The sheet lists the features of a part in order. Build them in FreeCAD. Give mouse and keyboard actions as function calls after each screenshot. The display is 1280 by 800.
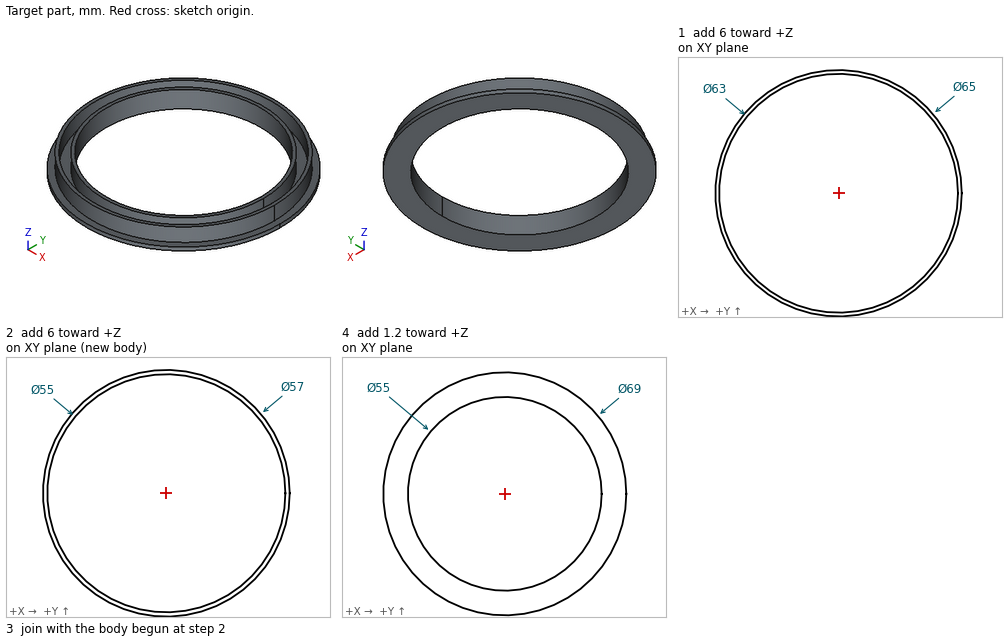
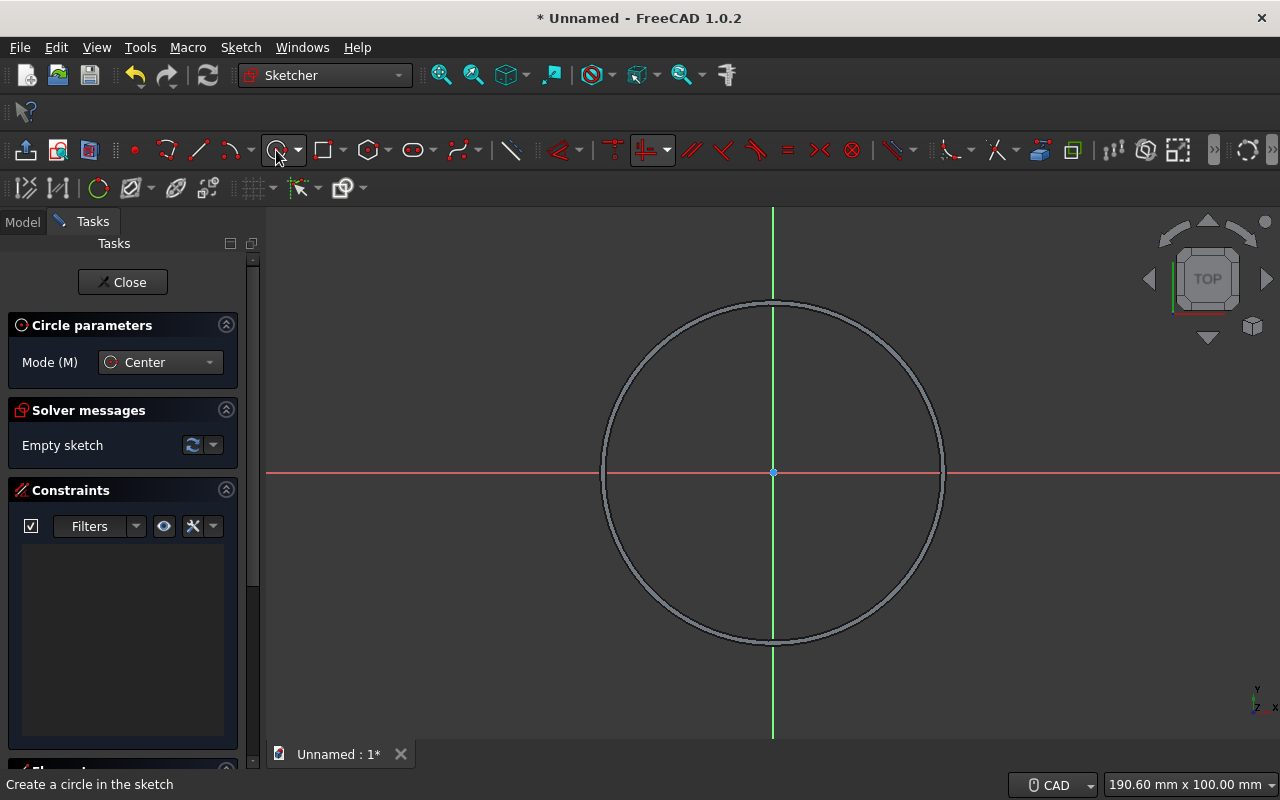
click(773, 473)
move(880, 366)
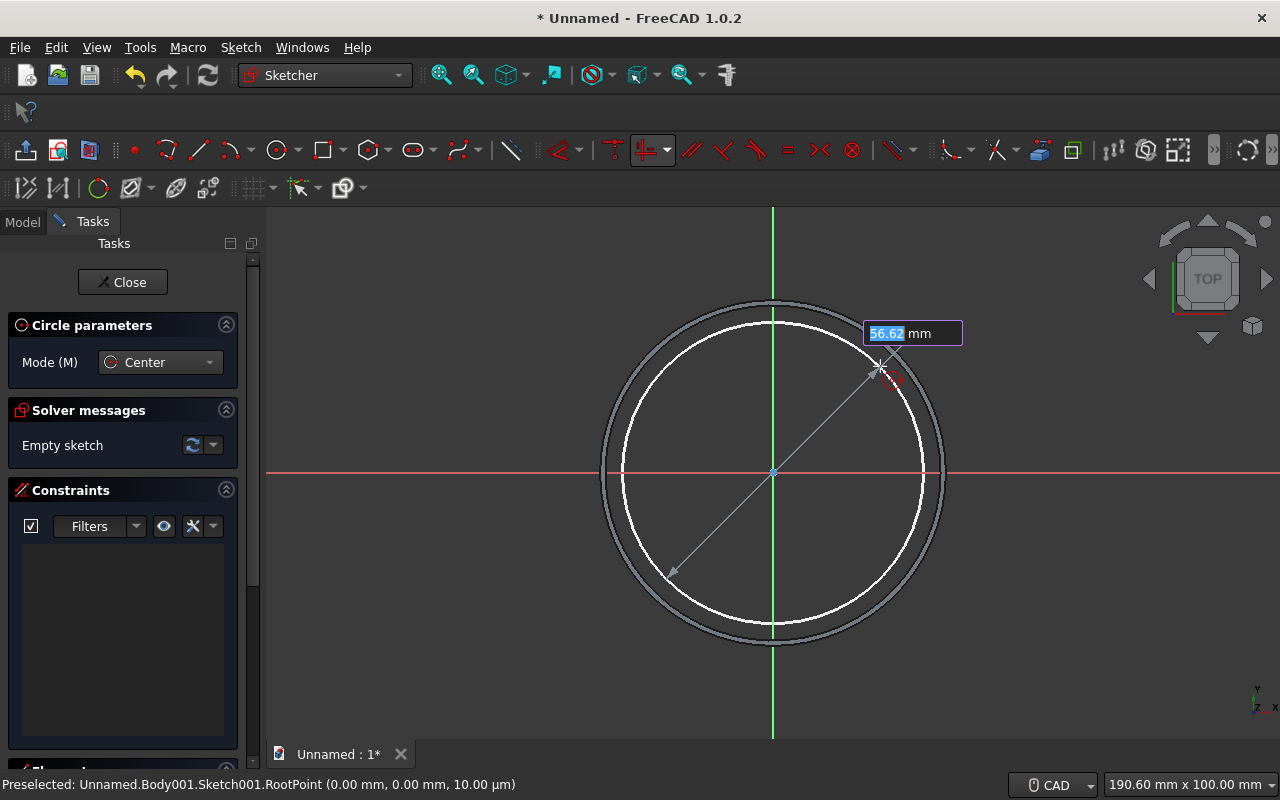
text(57)
key(Return)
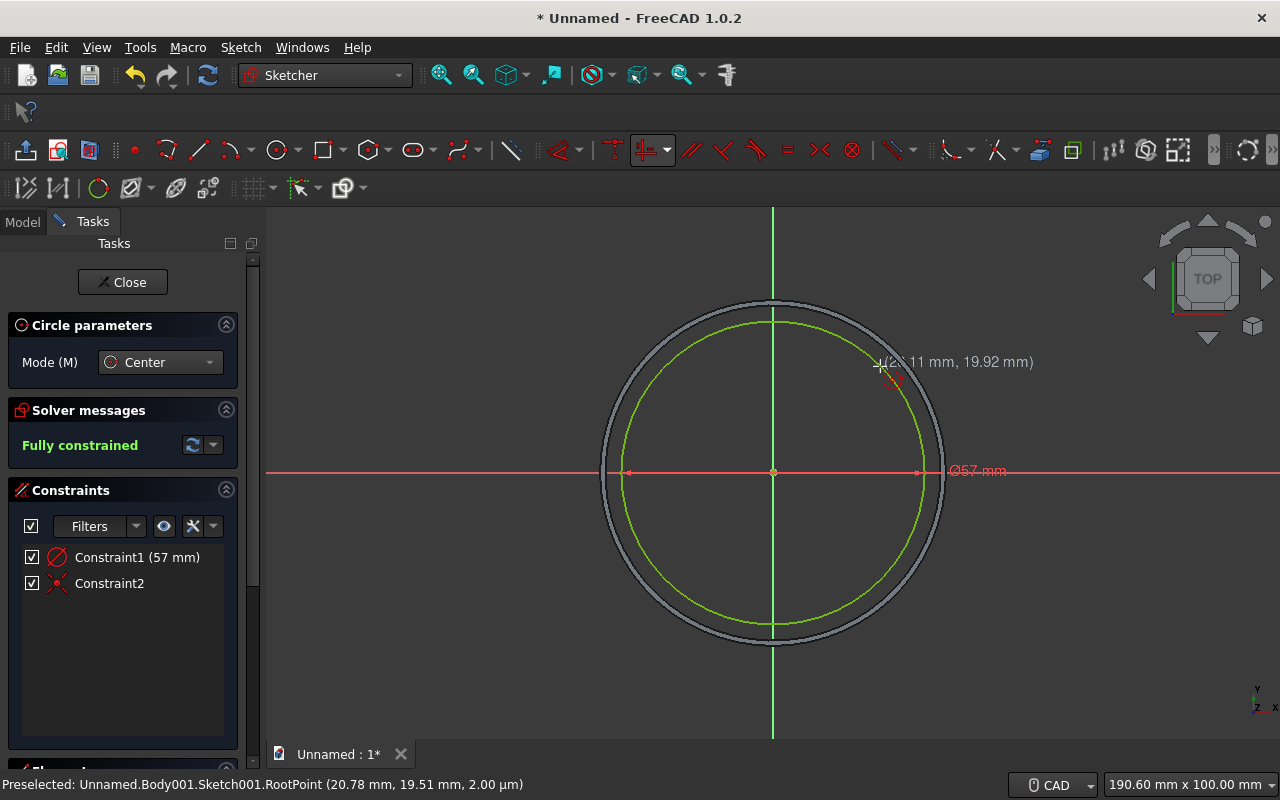
click(773, 473)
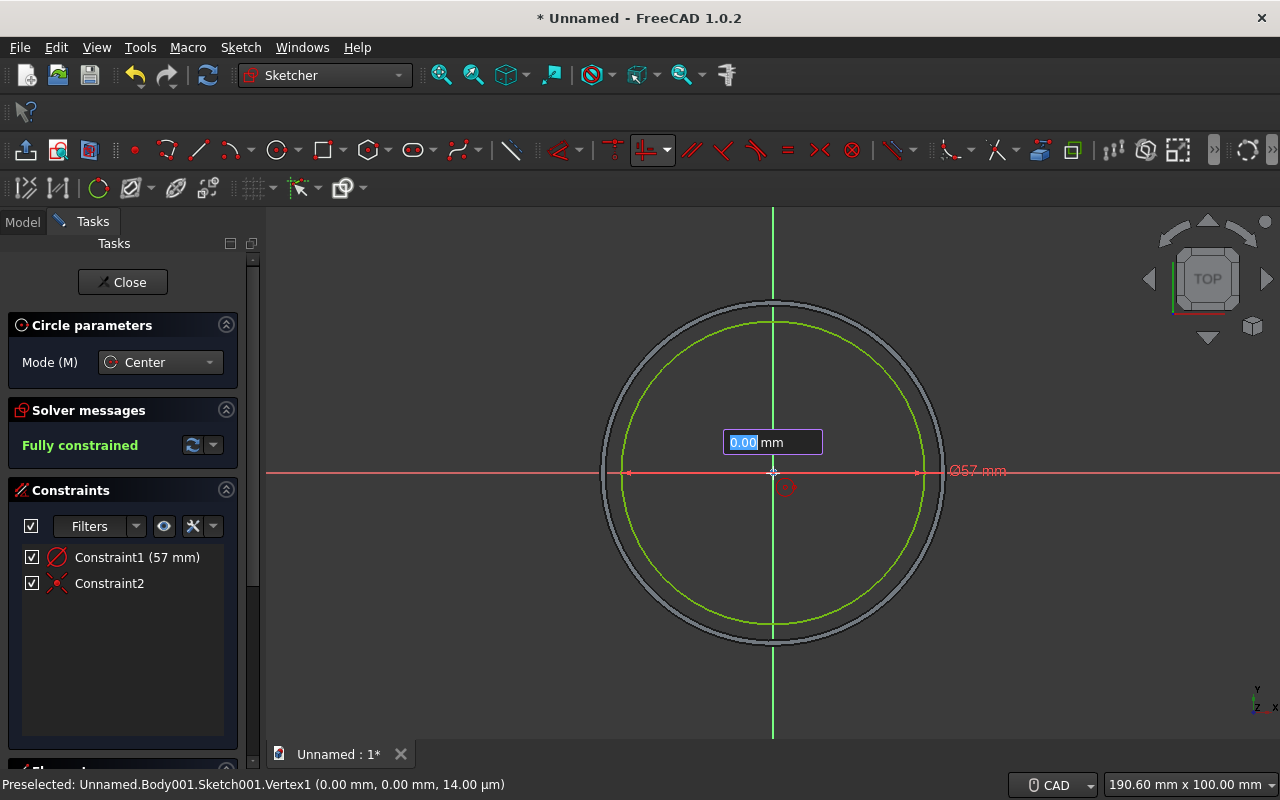
scroll(876, 370, up, 6)
move(876, 368)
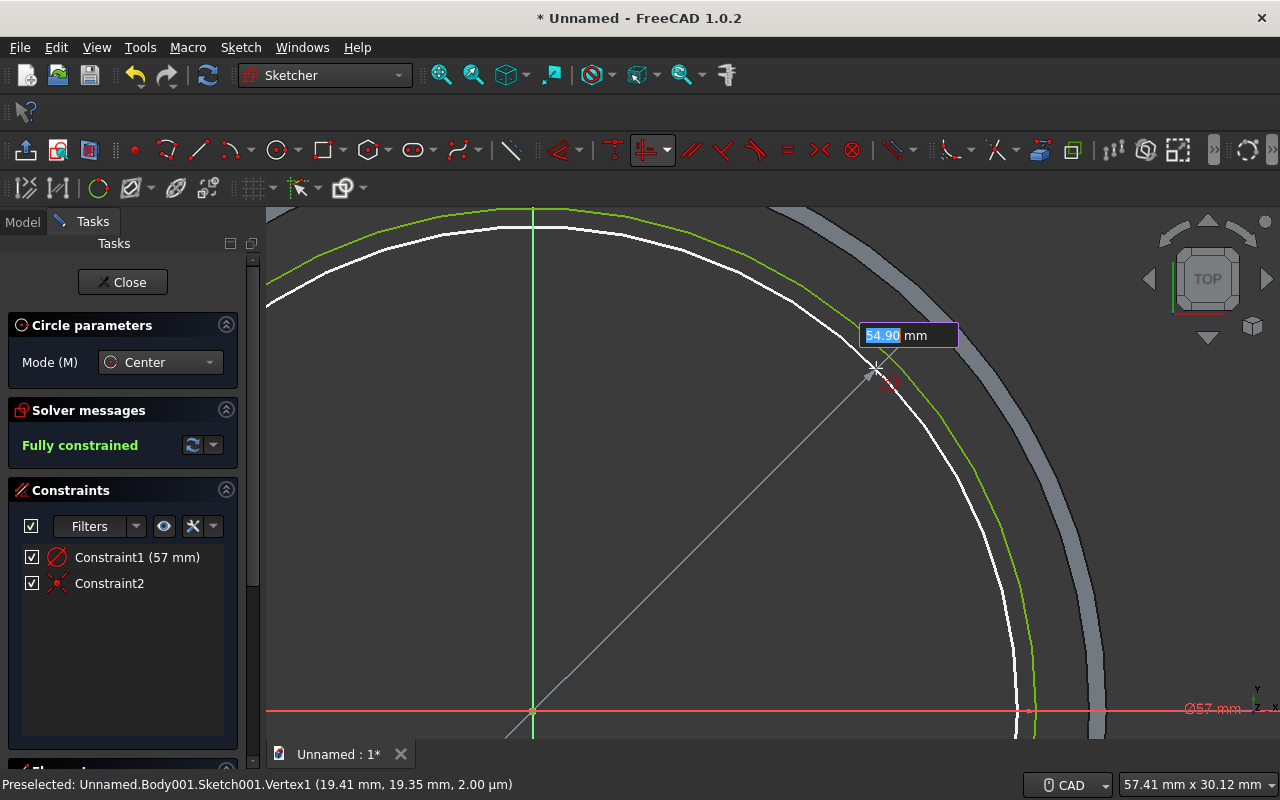
text(55)
key(Return)
key(Escape)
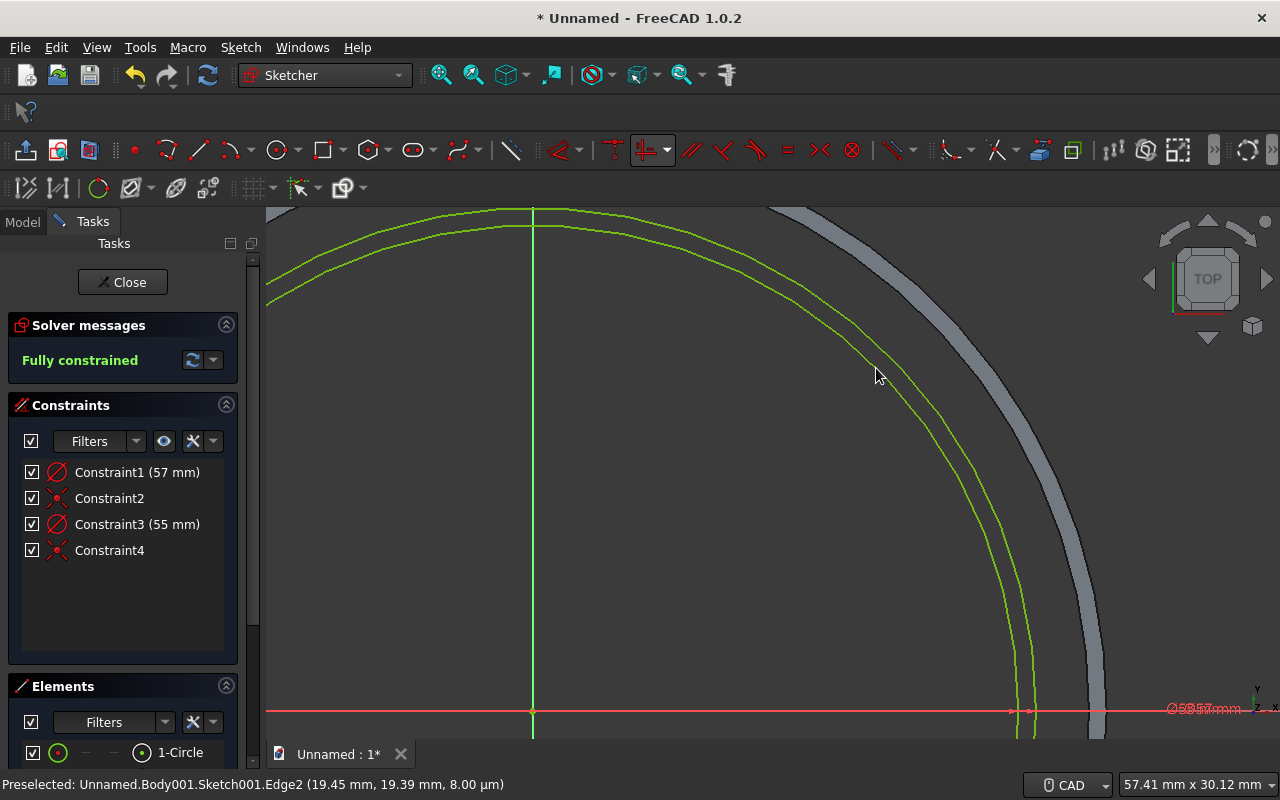
click(123, 282)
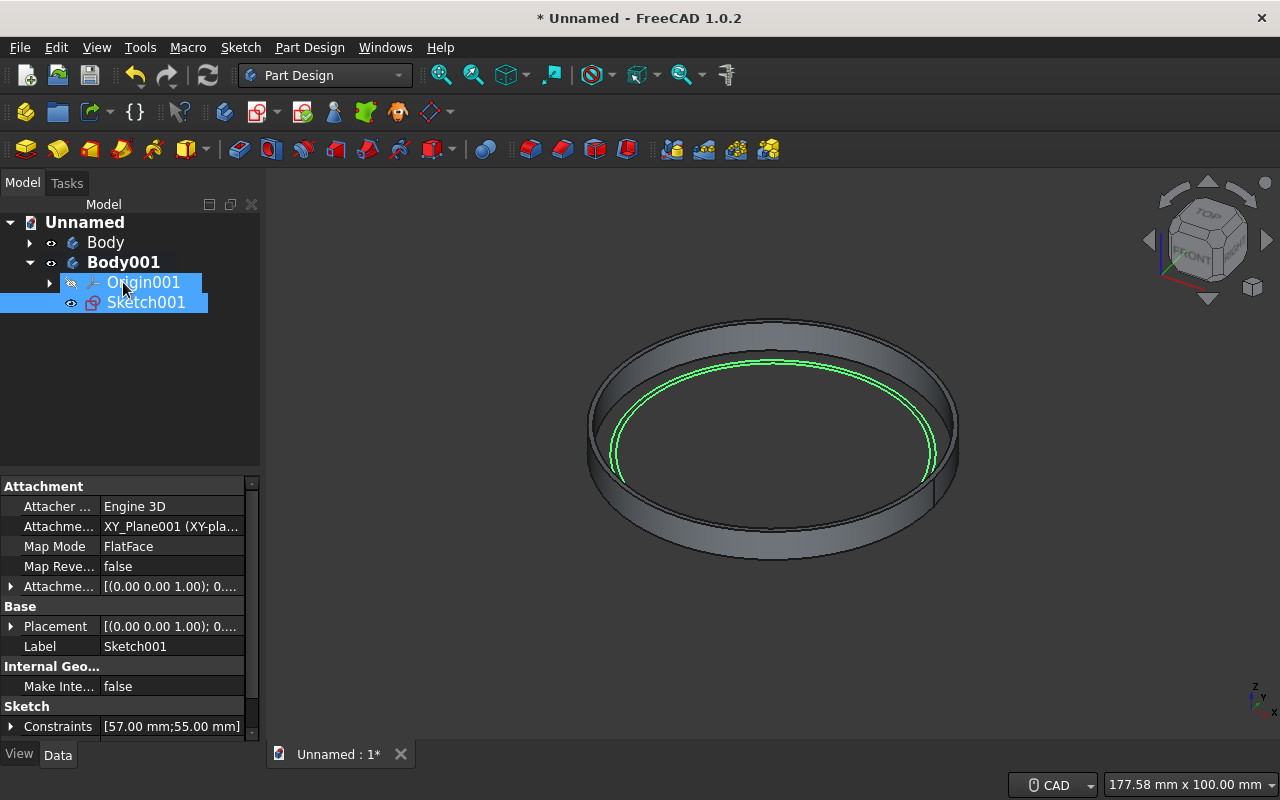
click(26, 150)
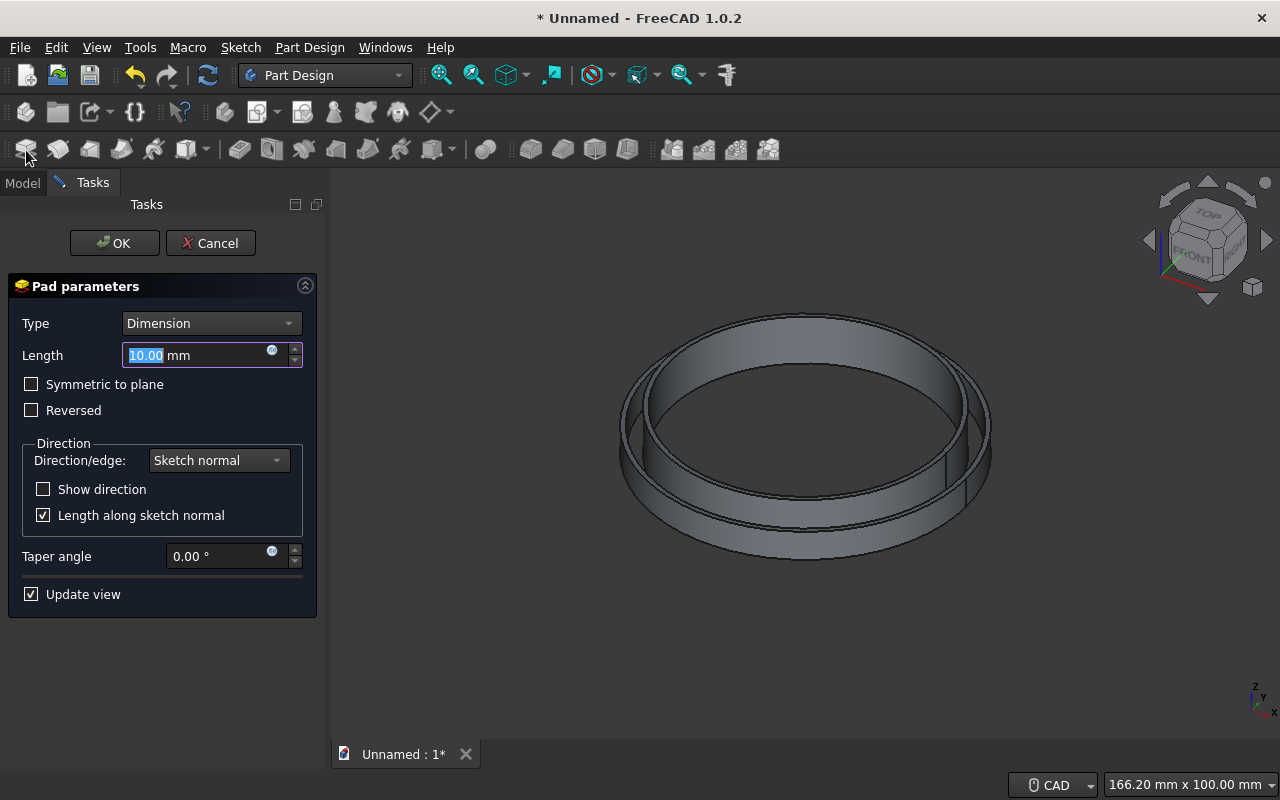
text(6)
key(Tab)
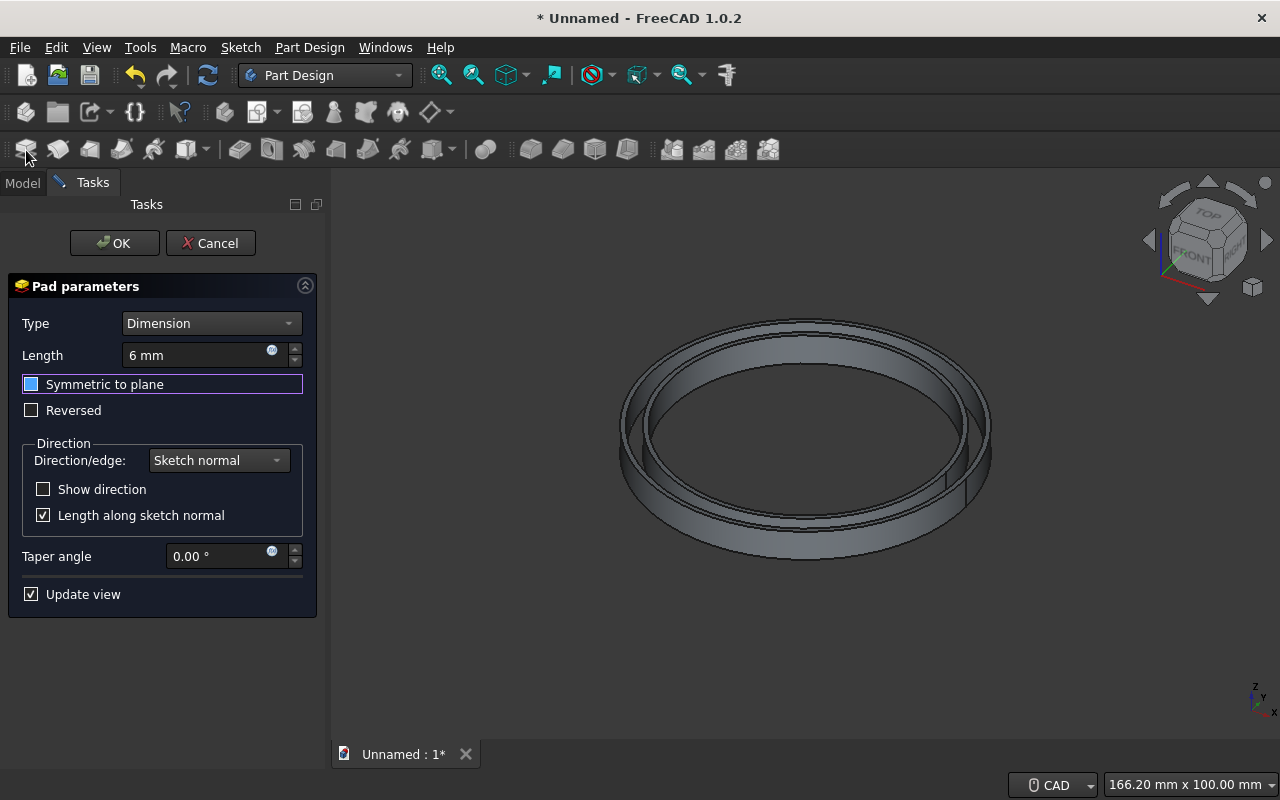
click(115, 243)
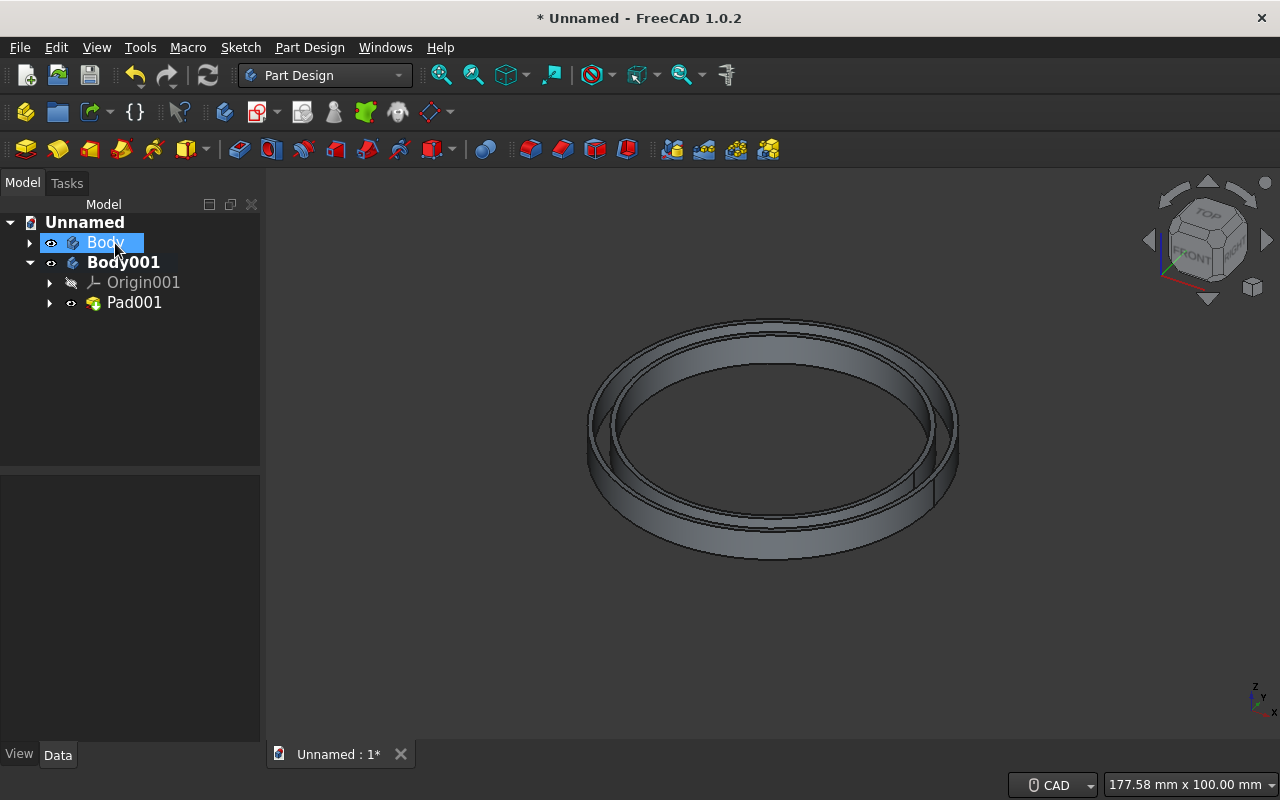
double_click(96, 243)